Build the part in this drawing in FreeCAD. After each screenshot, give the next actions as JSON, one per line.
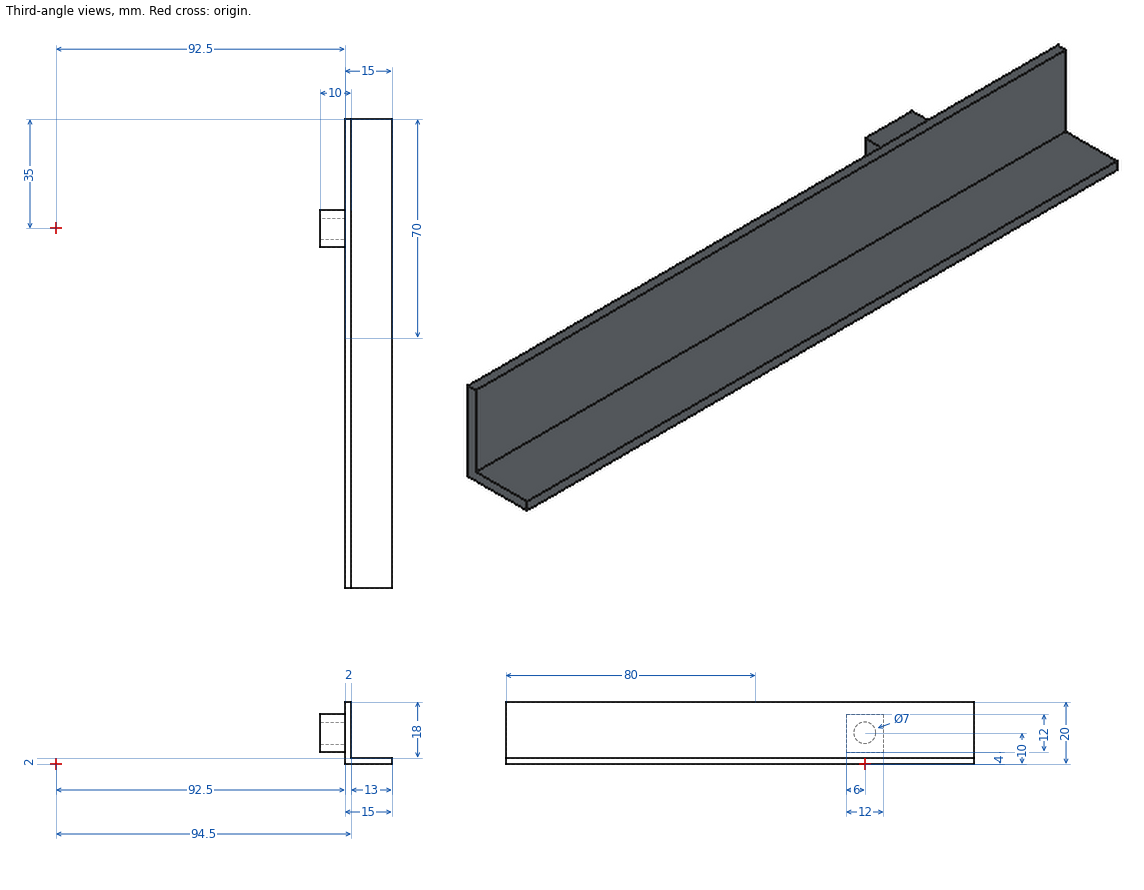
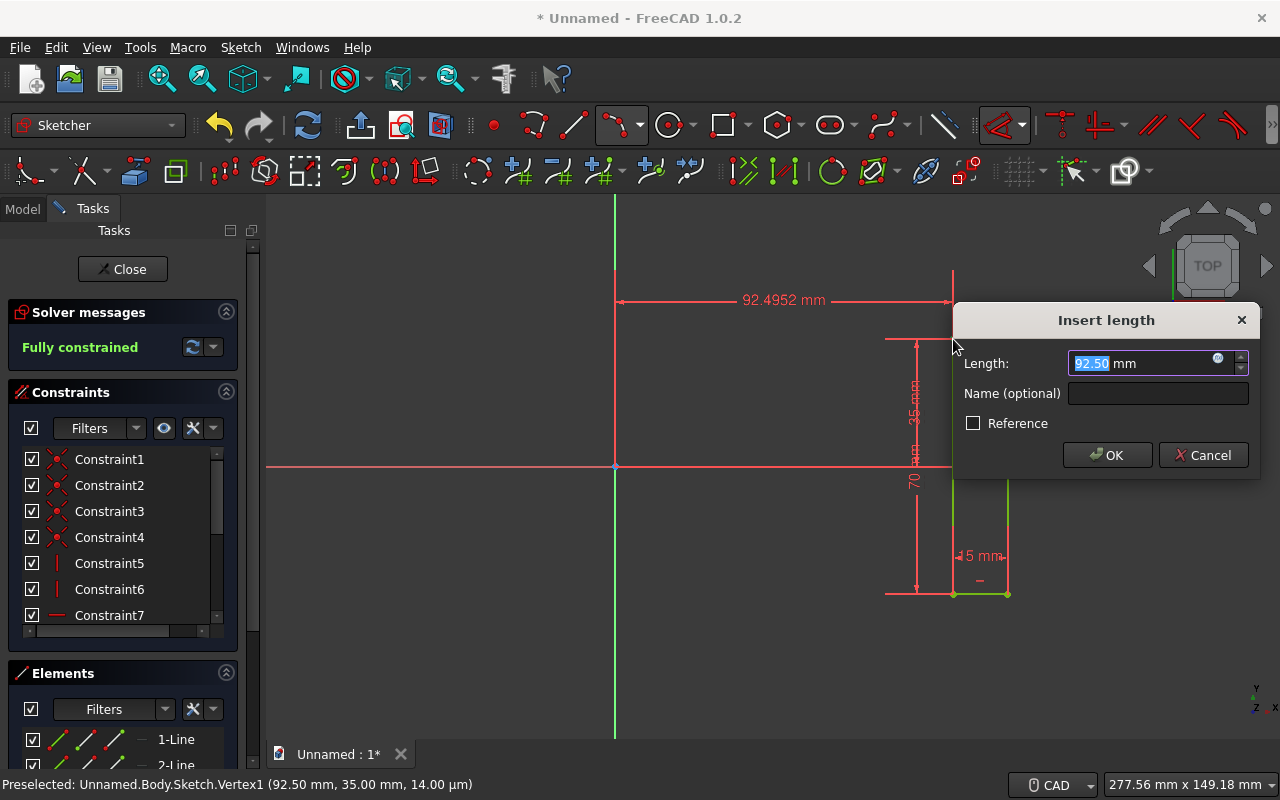
{"action": "type", "text": "92.5"}
{"action": "key", "text": "Return"}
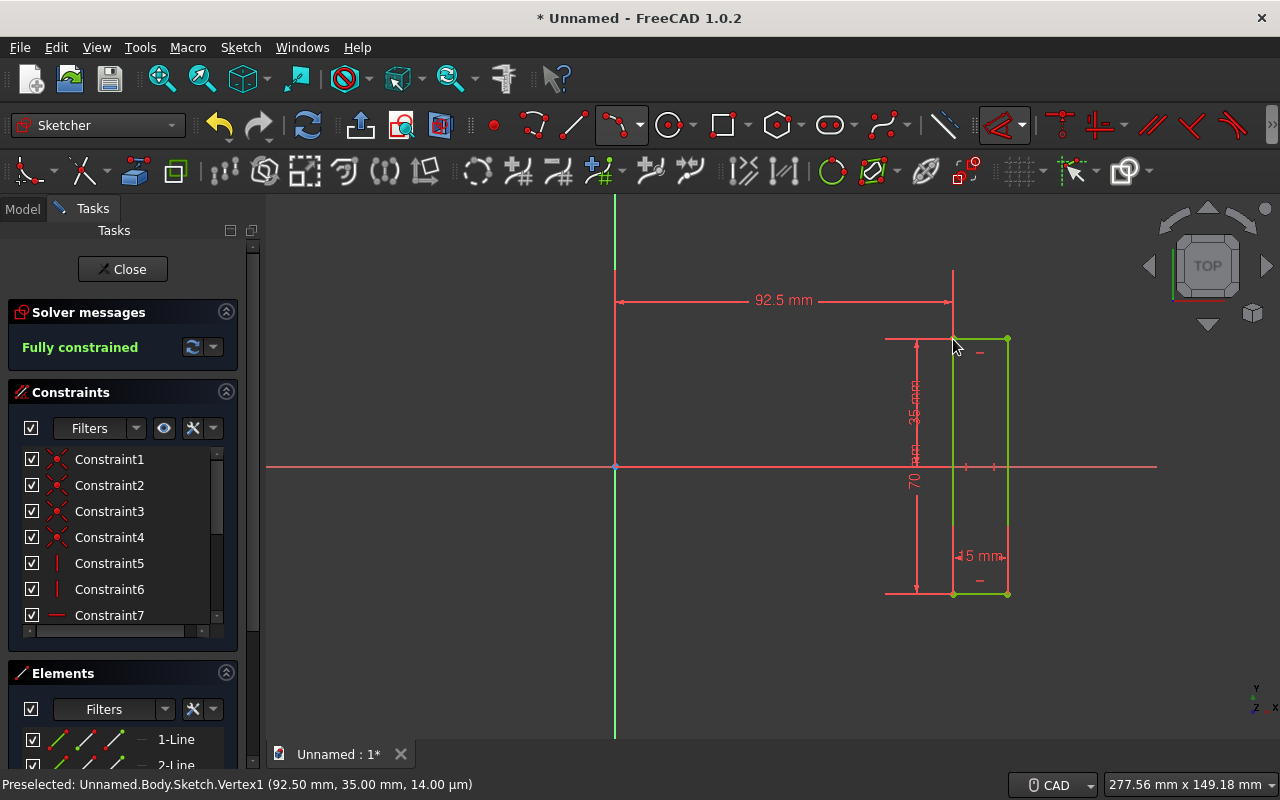
{"action": "left_click", "coordinate": [123, 269]}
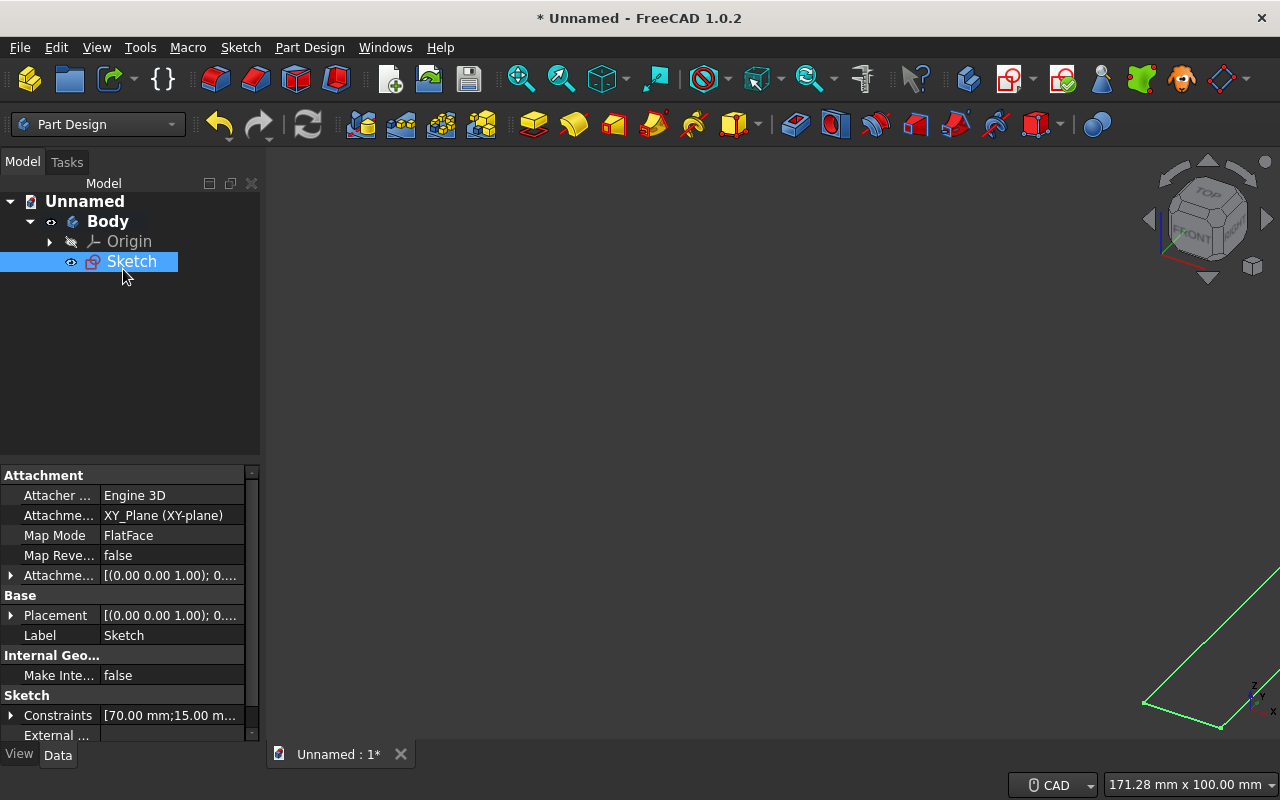
{"action": "left_click", "coordinate": [534, 124]}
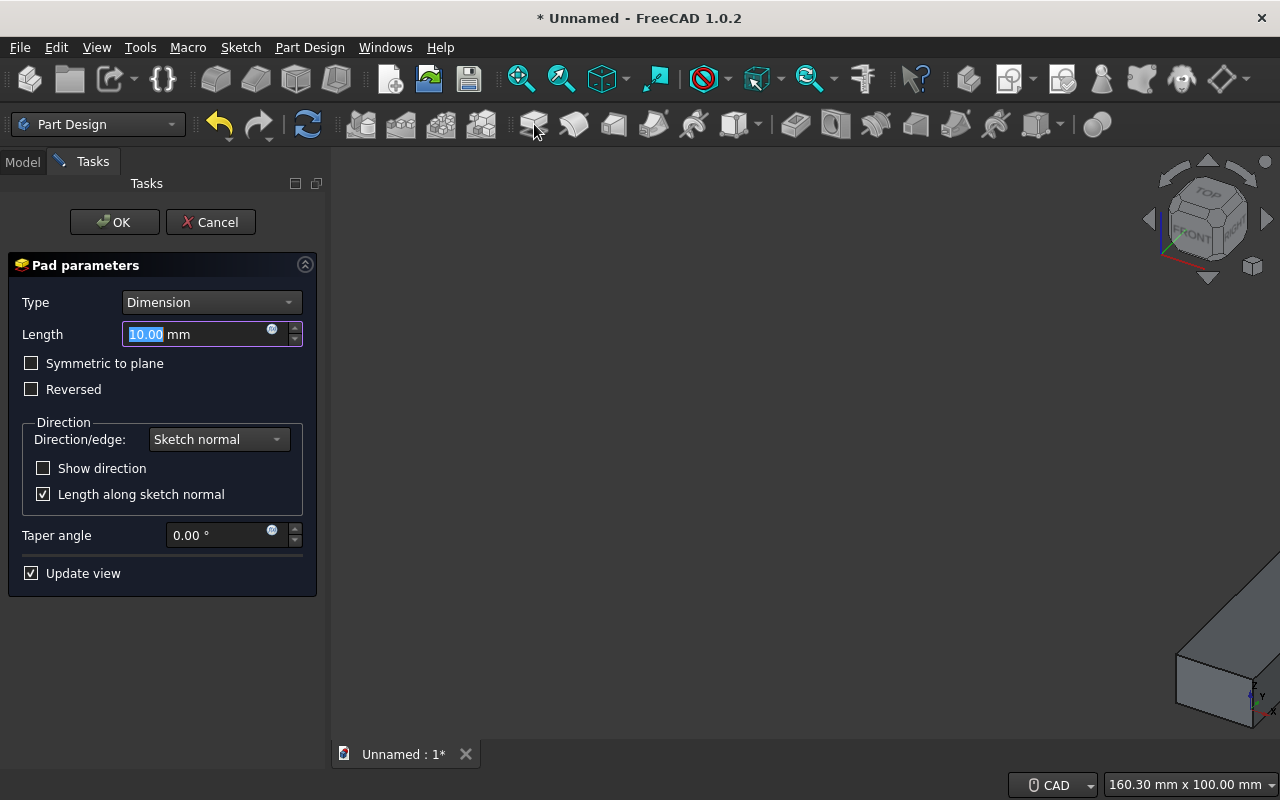
{"action": "type", "text": "20"}
{"action": "key", "text": "Tab"}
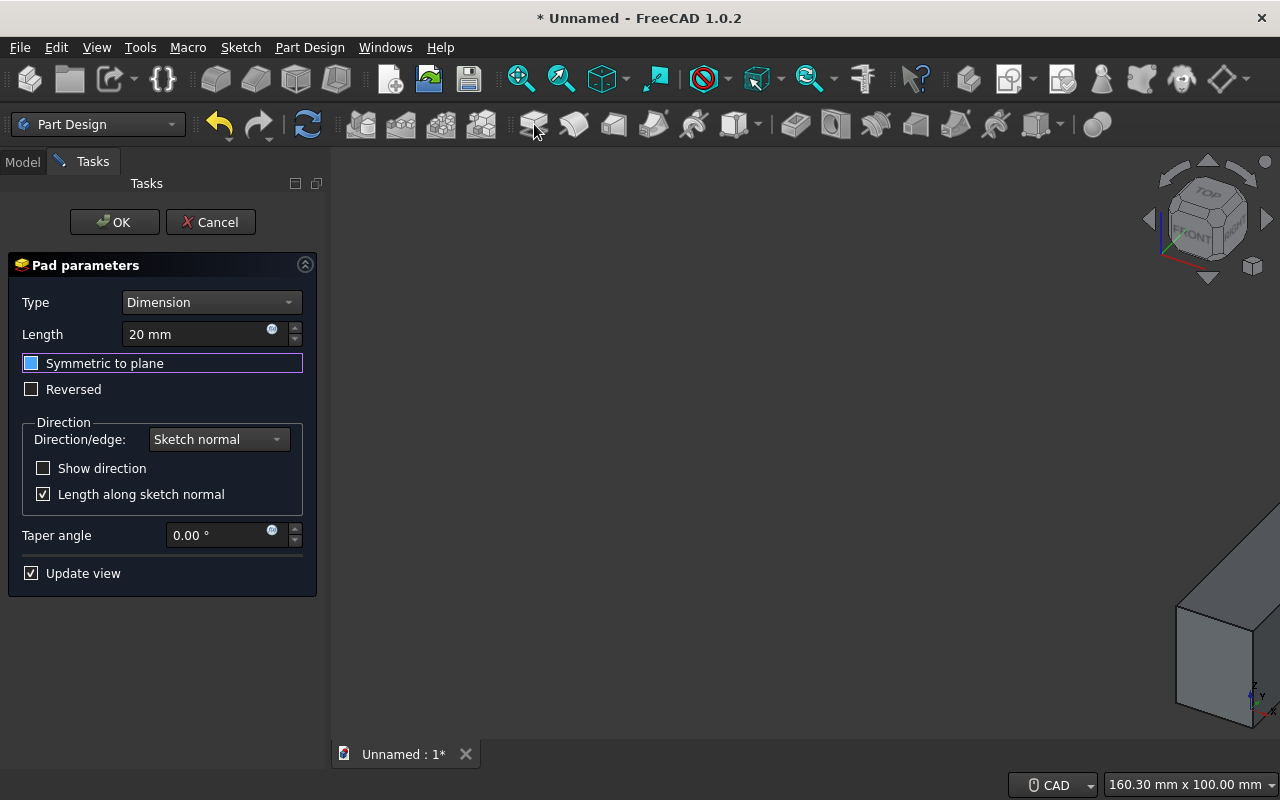
{"action": "left_click", "coordinate": [115, 222]}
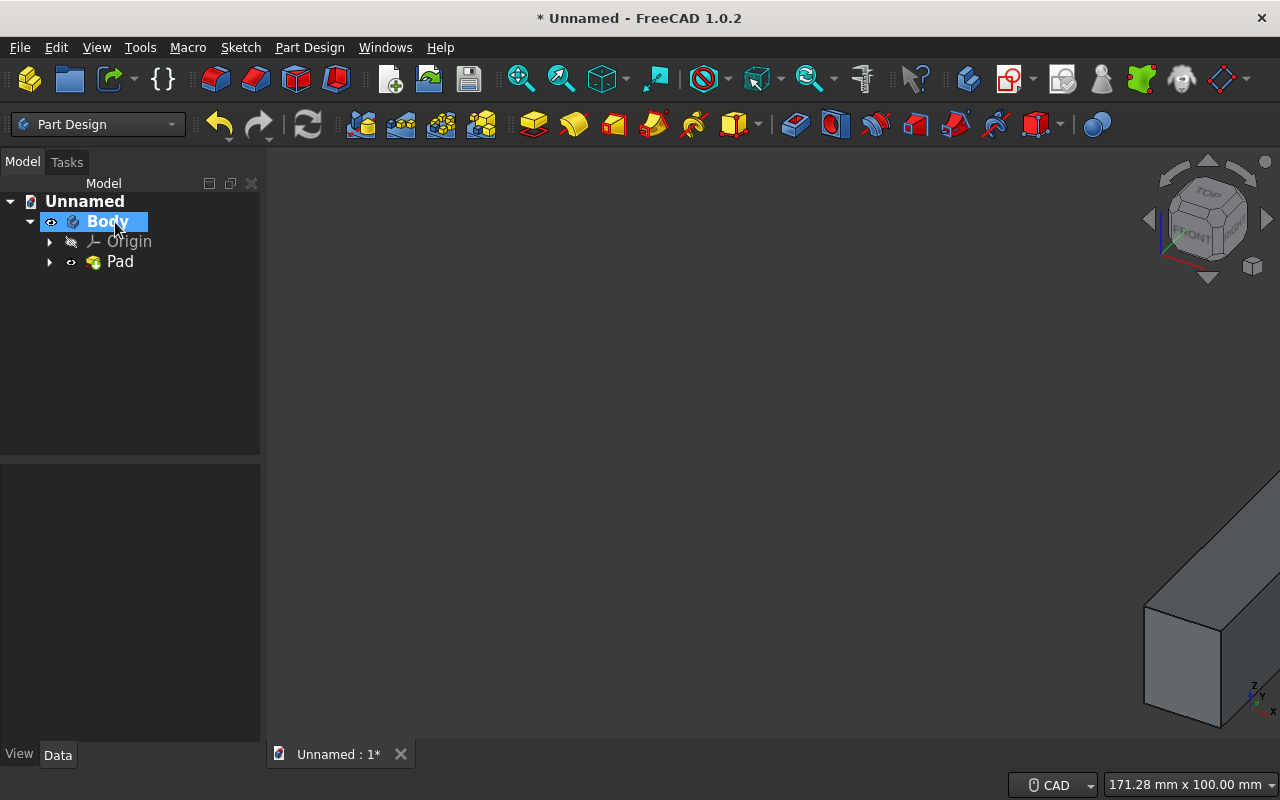
{"action": "left_click", "coordinate": [522, 80]}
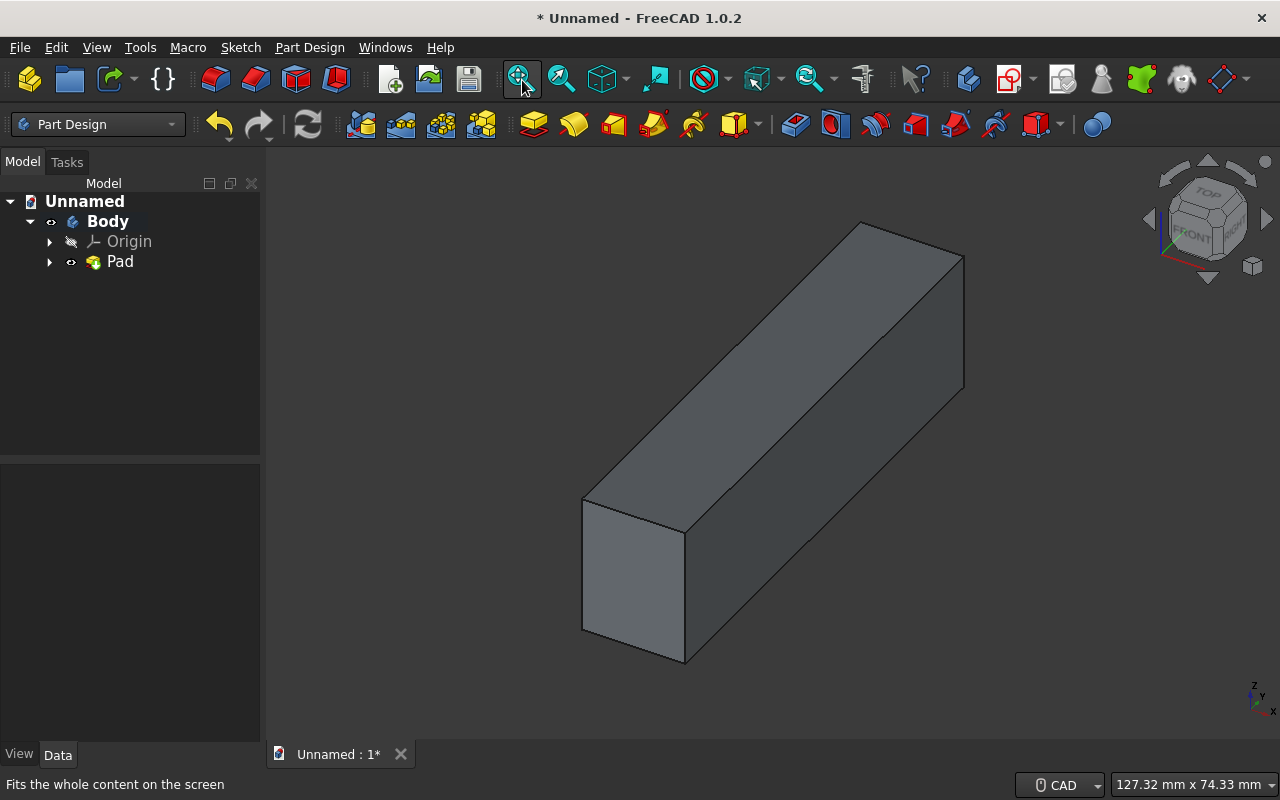
{"action": "left_click", "coordinate": [634, 580]}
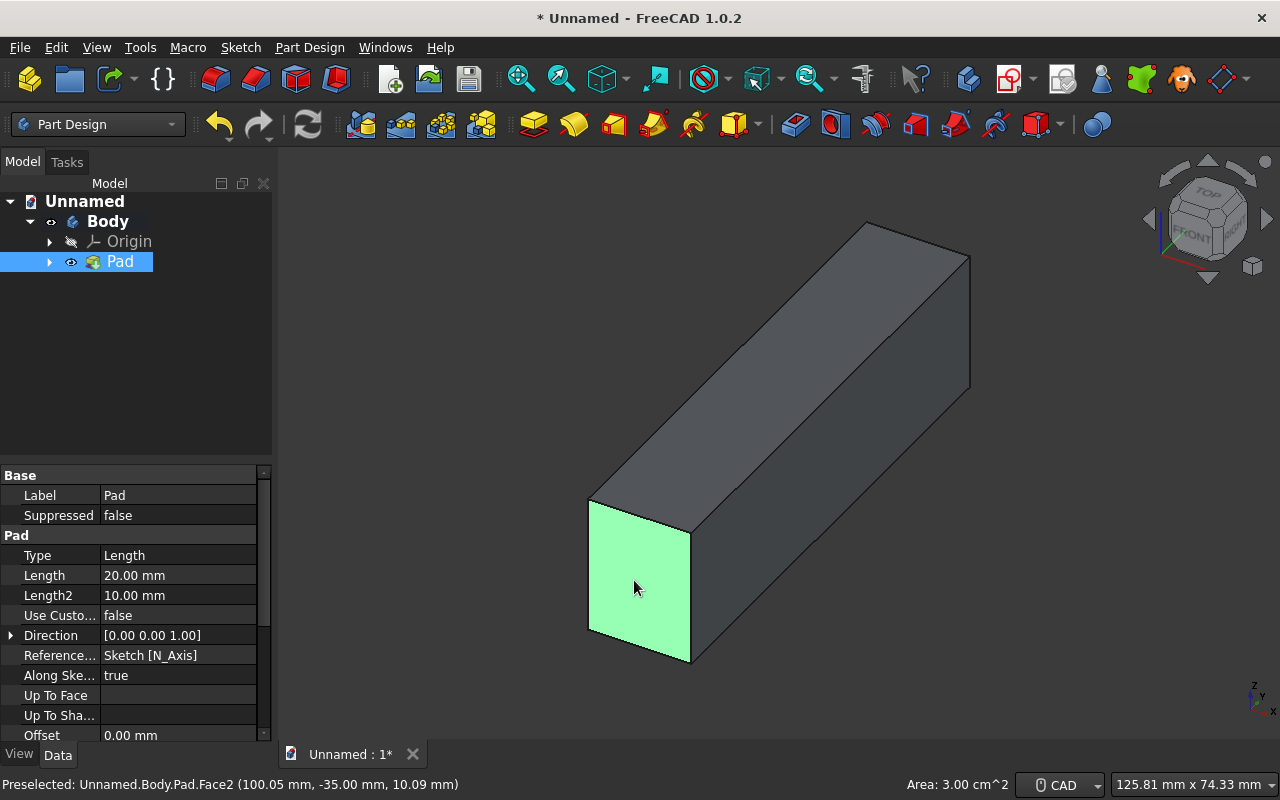
{"action": "left_click", "coordinate": [1010, 80]}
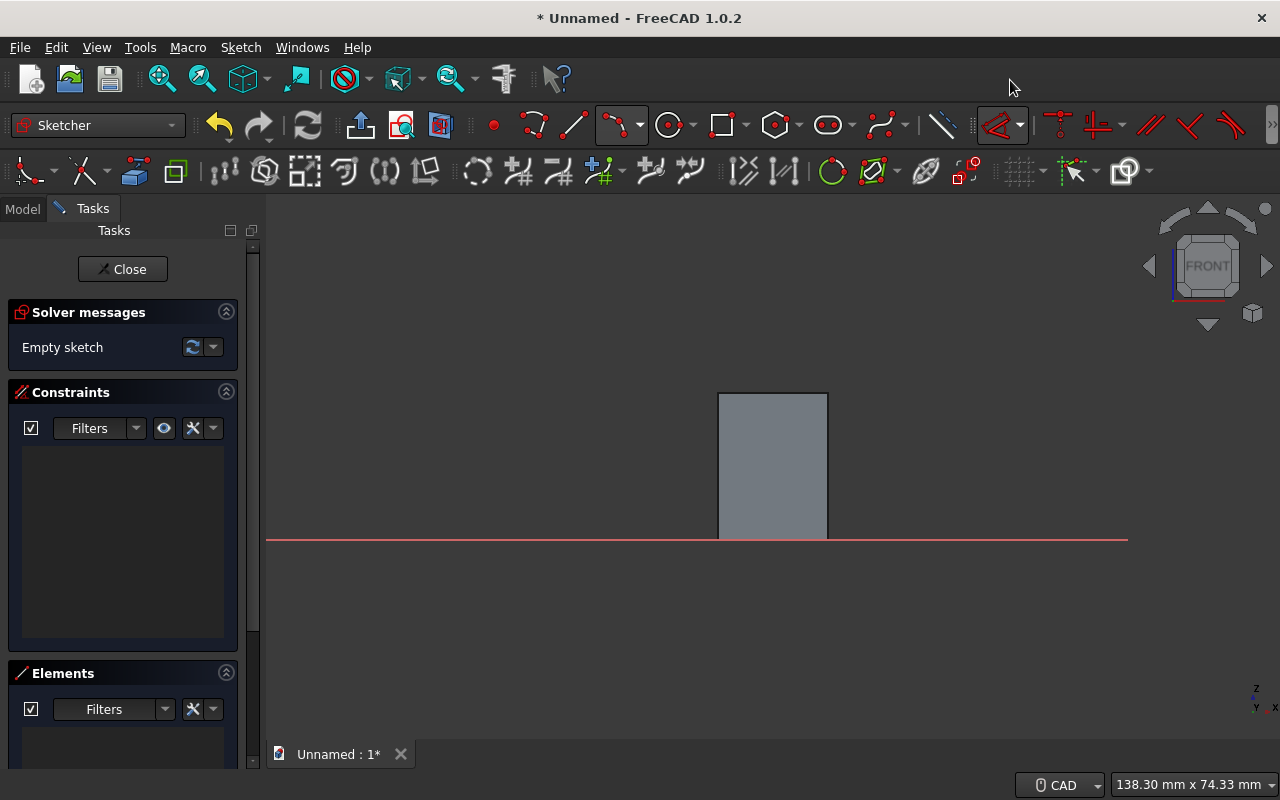
{"action": "scroll", "coordinate": [824, 455], "scroll_direction": "up", "scroll_amount": 5}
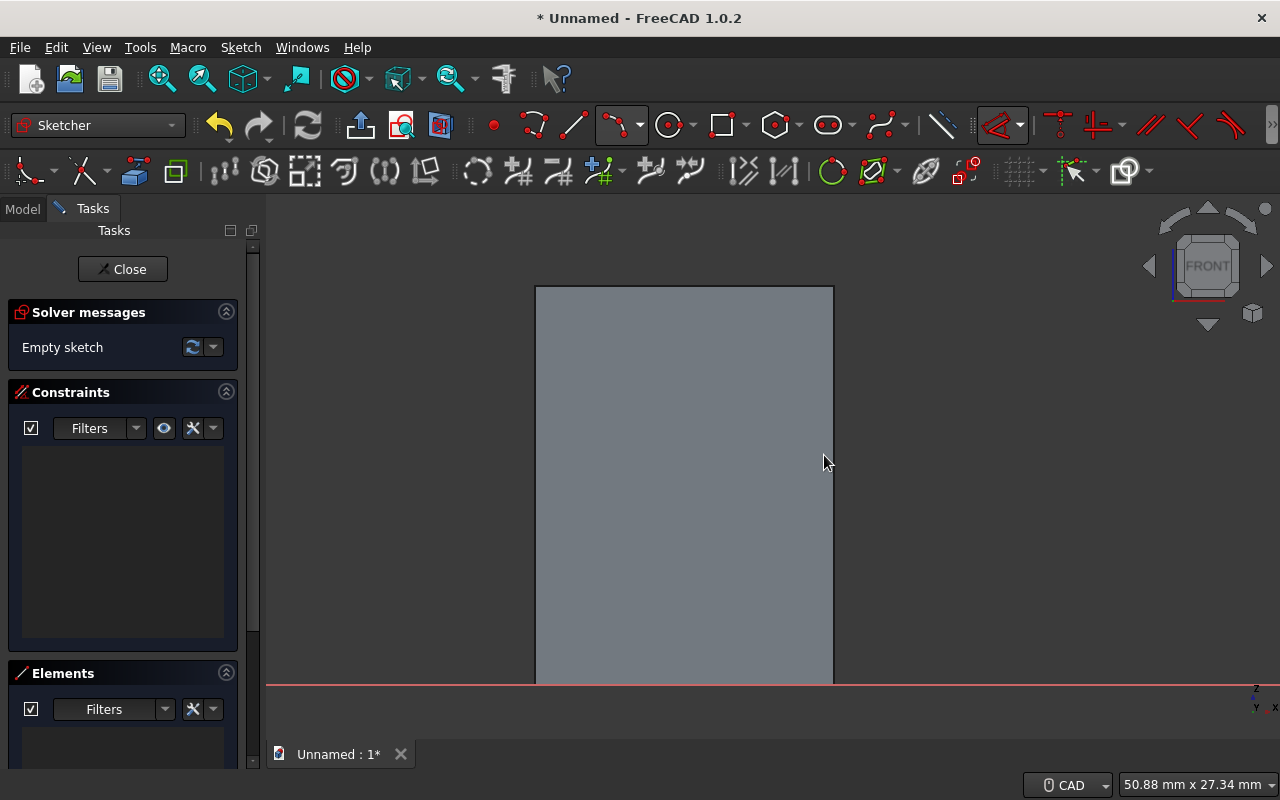
{"action": "left_click", "coordinate": [722, 126]}